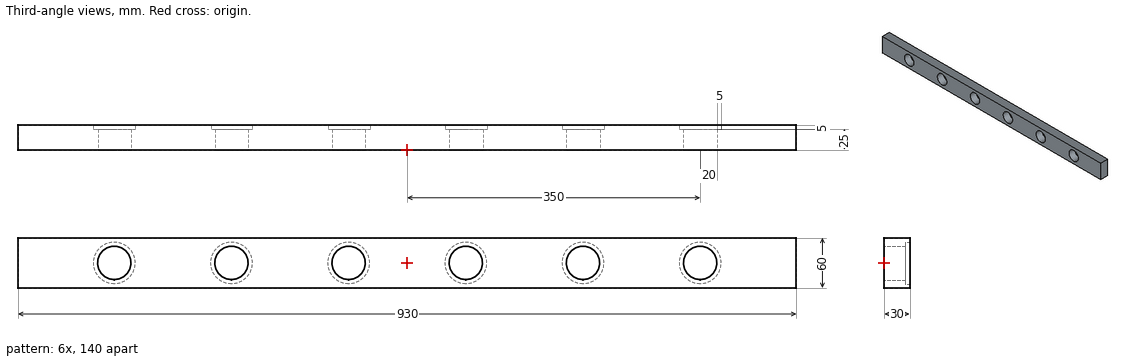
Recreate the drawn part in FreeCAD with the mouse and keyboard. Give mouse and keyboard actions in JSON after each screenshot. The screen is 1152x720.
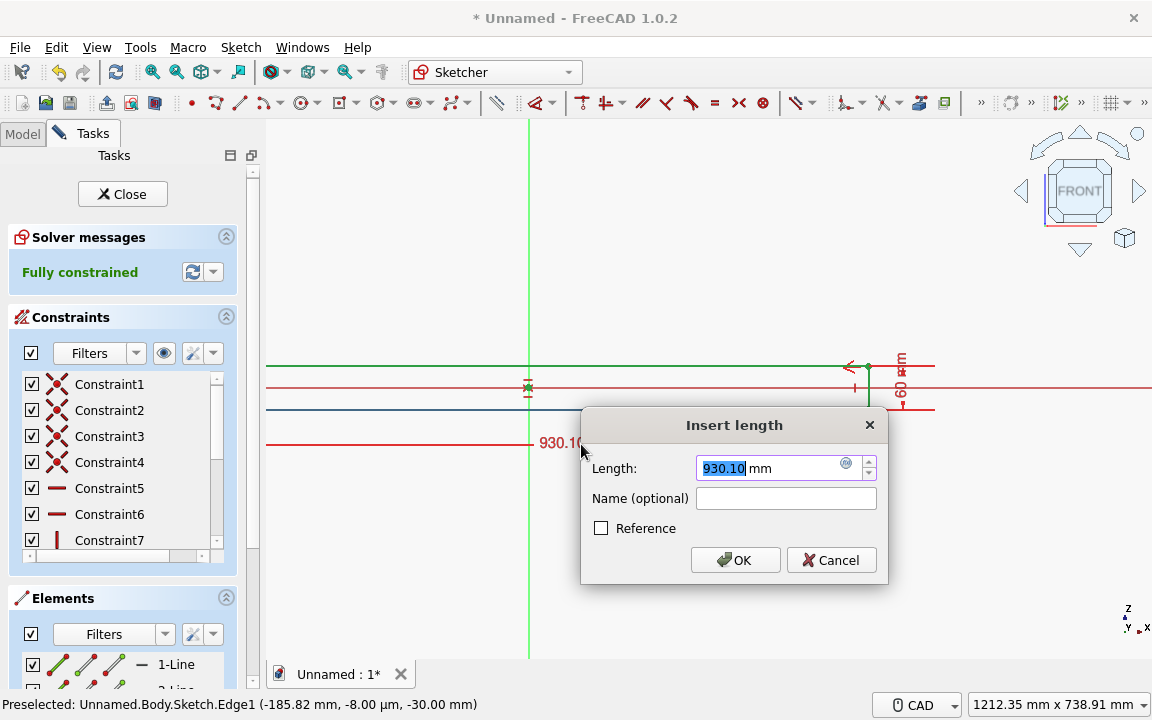
{"action": "type", "text": "930"}
{"action": "key", "text": "Return"}
{"action": "key", "text": "Escape"}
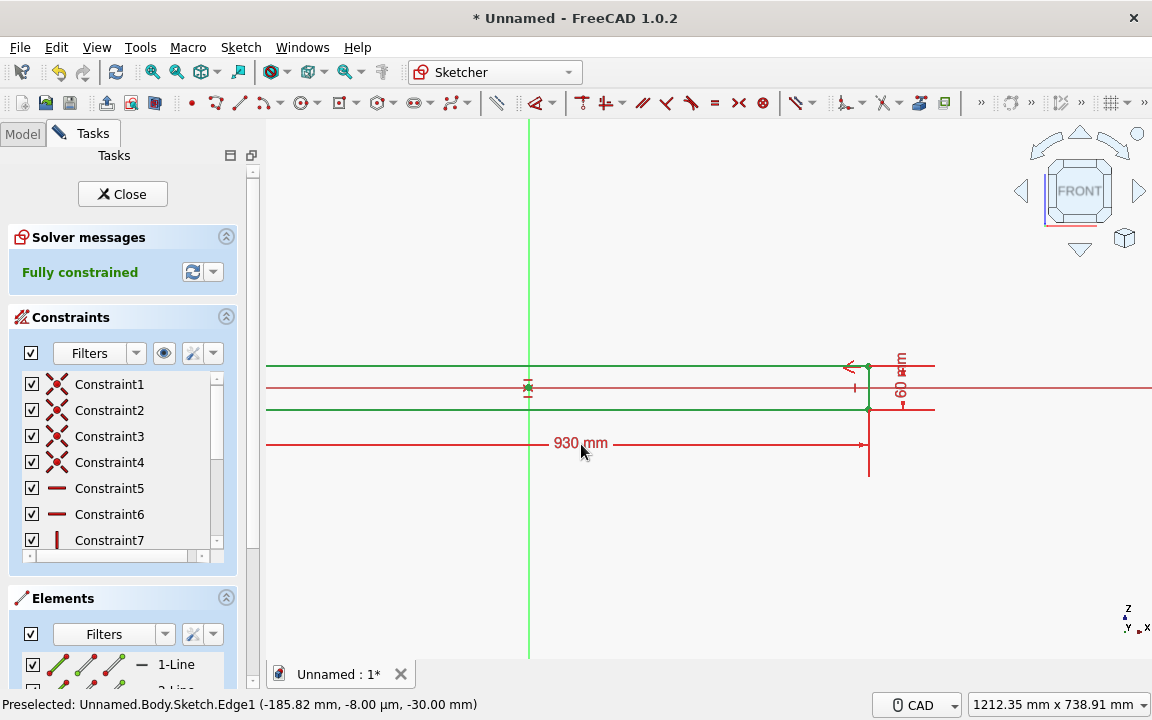
{"action": "left_click", "coordinate": [123, 194]}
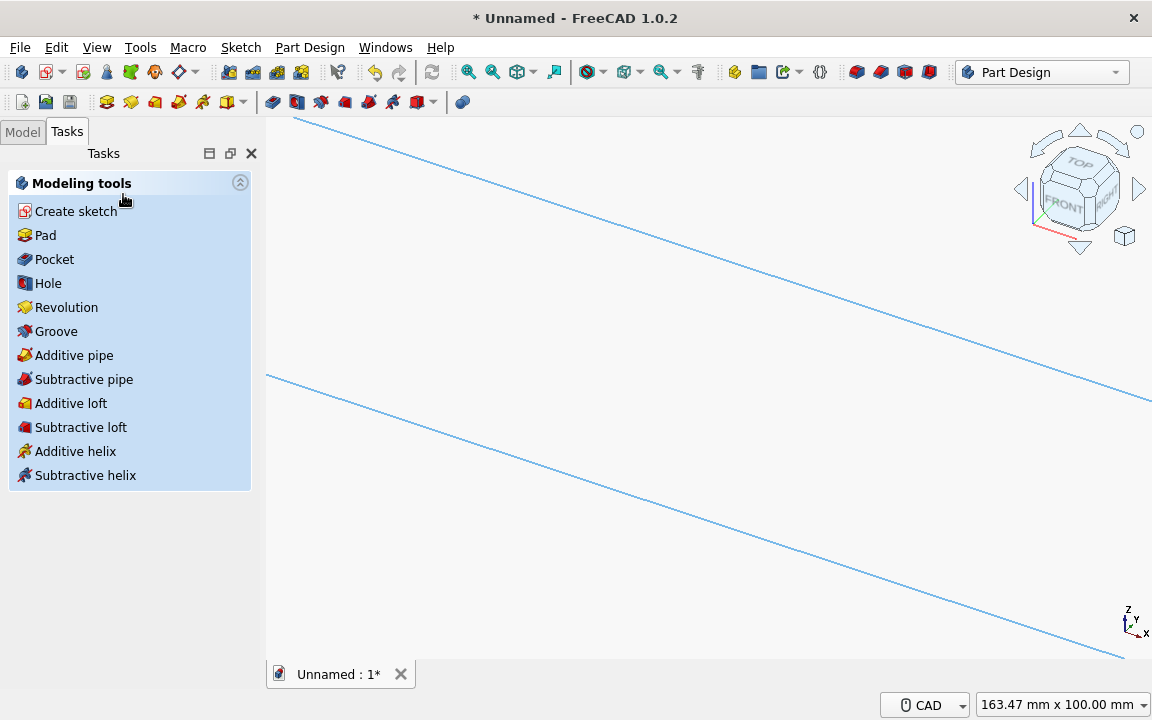
{"action": "left_click", "coordinate": [108, 102]}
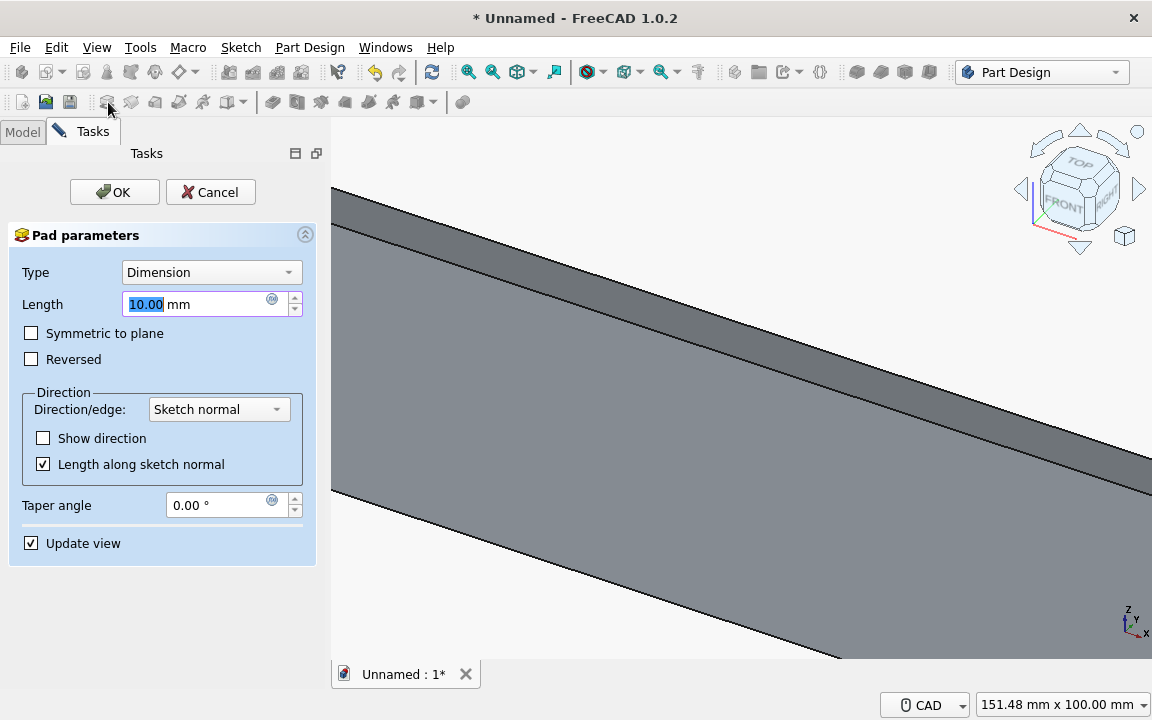
{"action": "type", "text": "30"}
{"action": "key", "text": "Tab"}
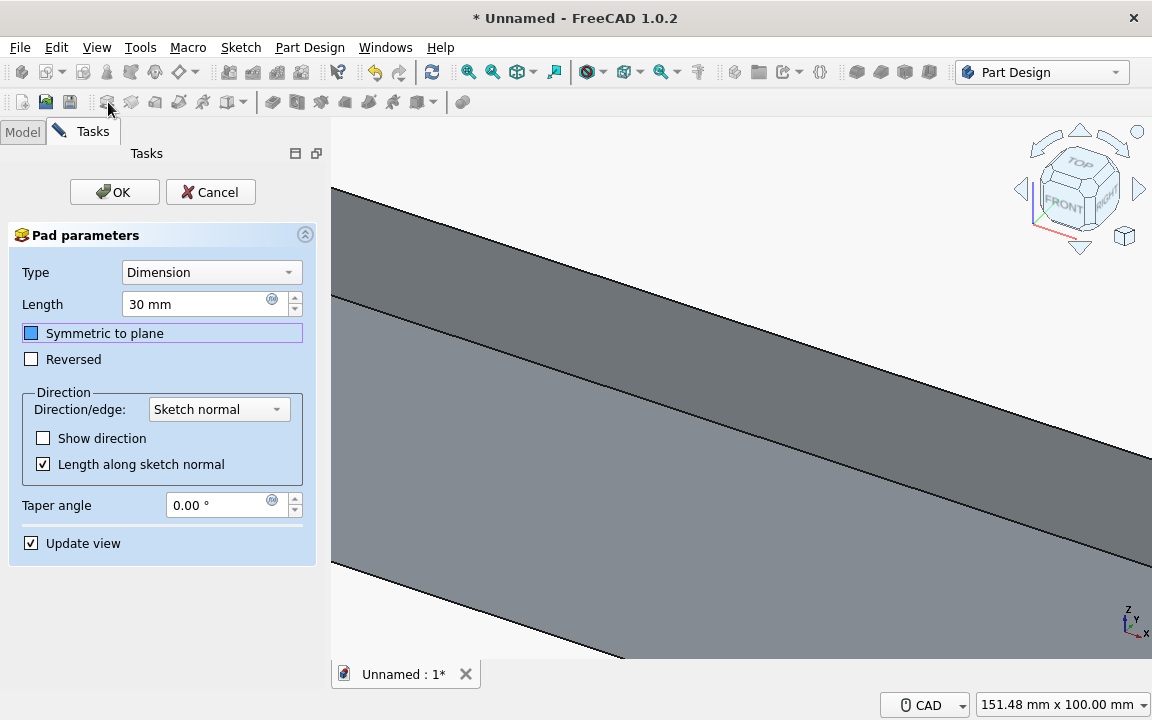
{"action": "left_click", "coordinate": [30, 359]}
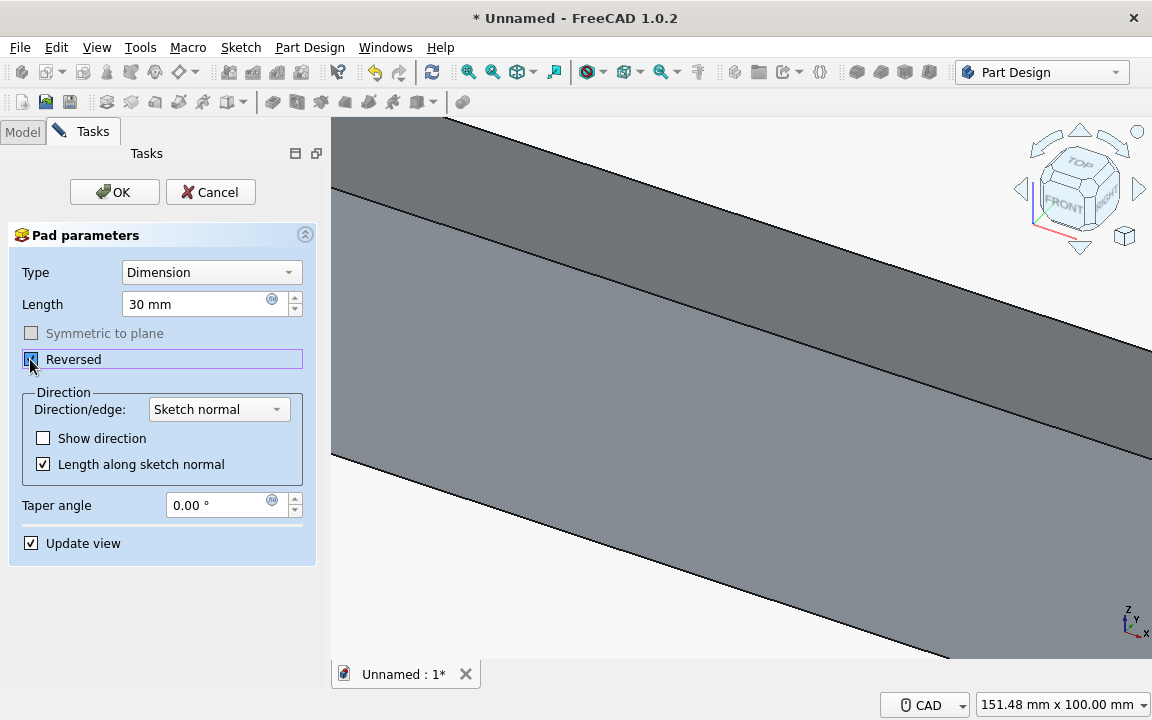
{"action": "left_click", "coordinate": [115, 192]}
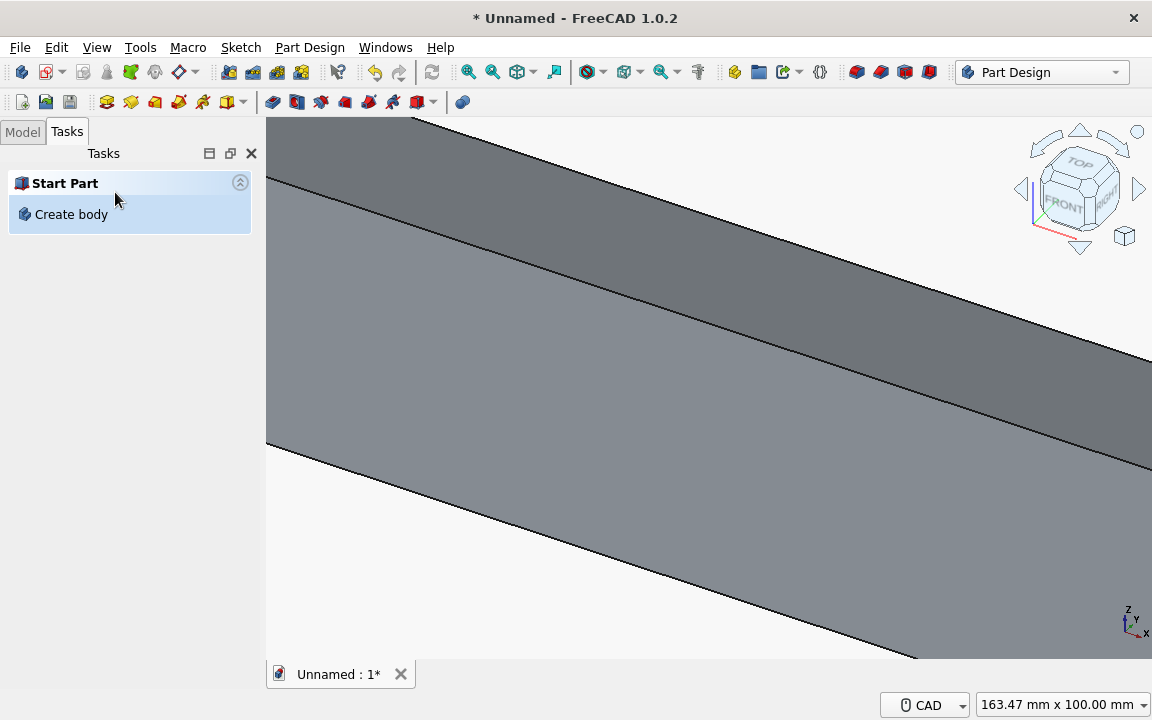
{"action": "left_click", "coordinate": [470, 72]}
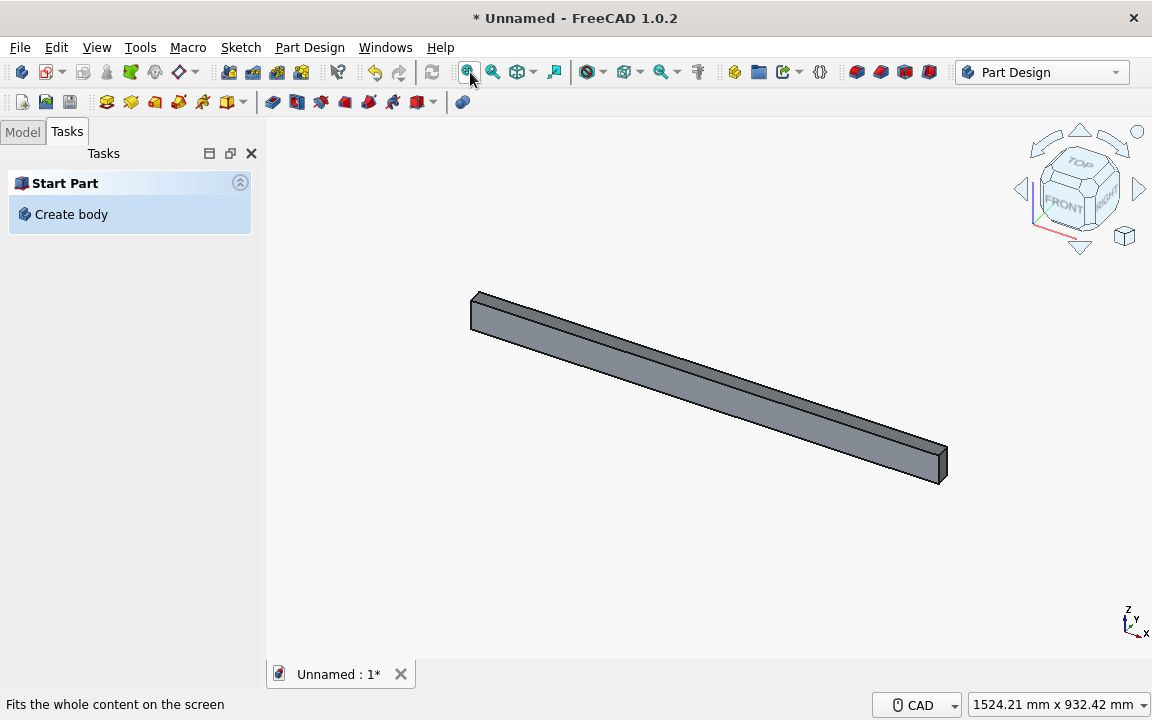
{"action": "left_click", "coordinate": [46, 72]}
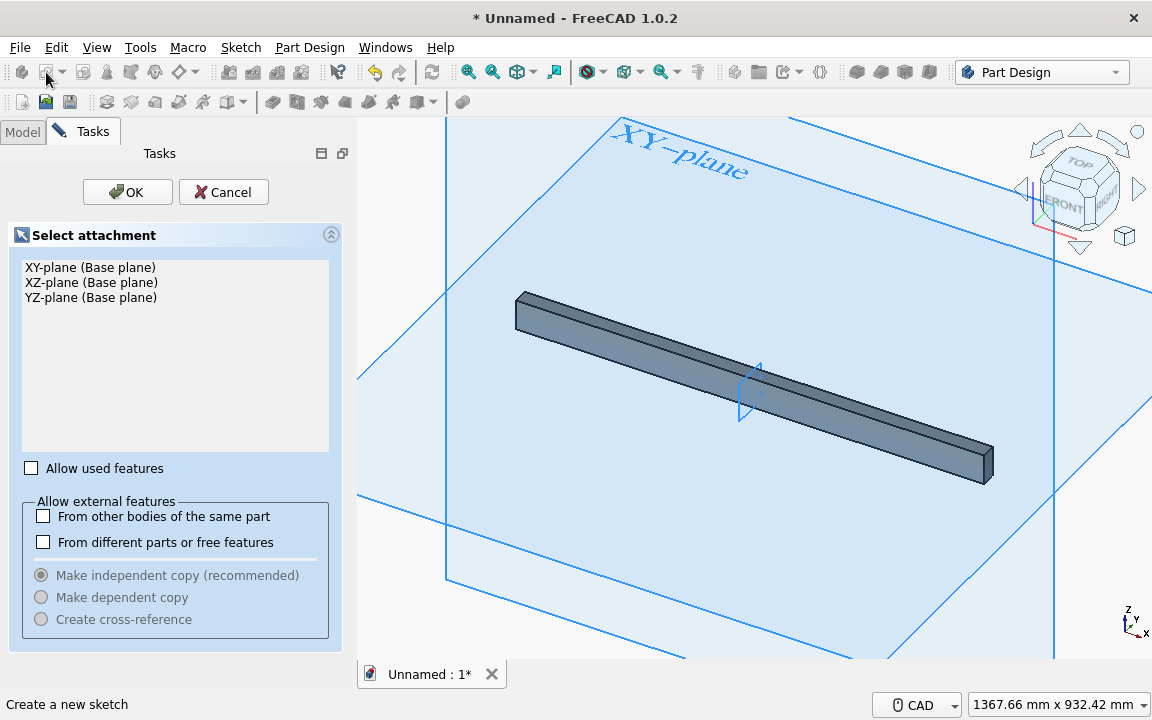
{"action": "left_click", "coordinate": [82, 268]}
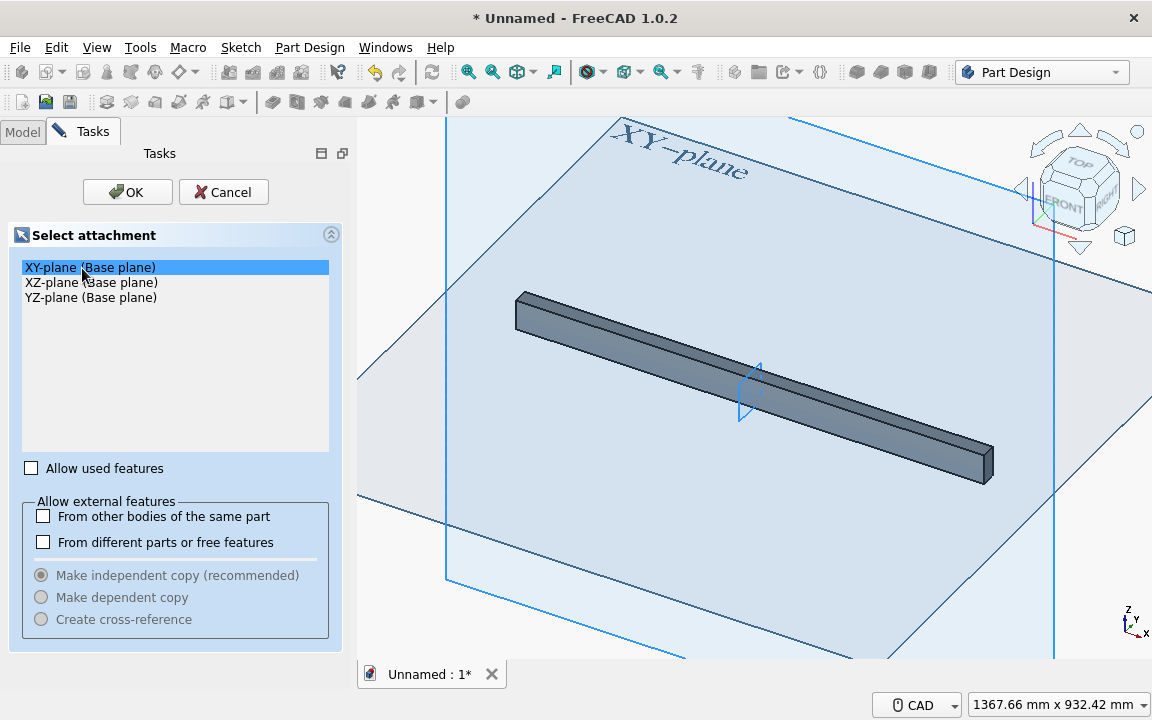
{"action": "left_click", "coordinate": [128, 192]}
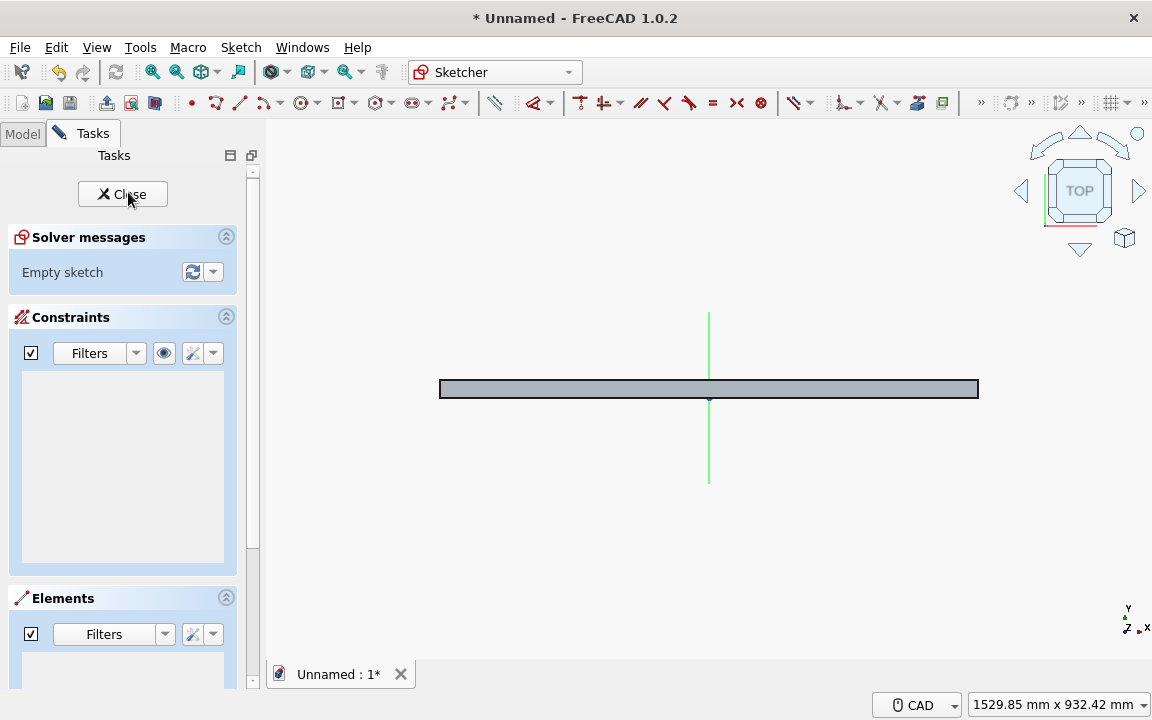
{"action": "left_click", "coordinate": [156, 104]}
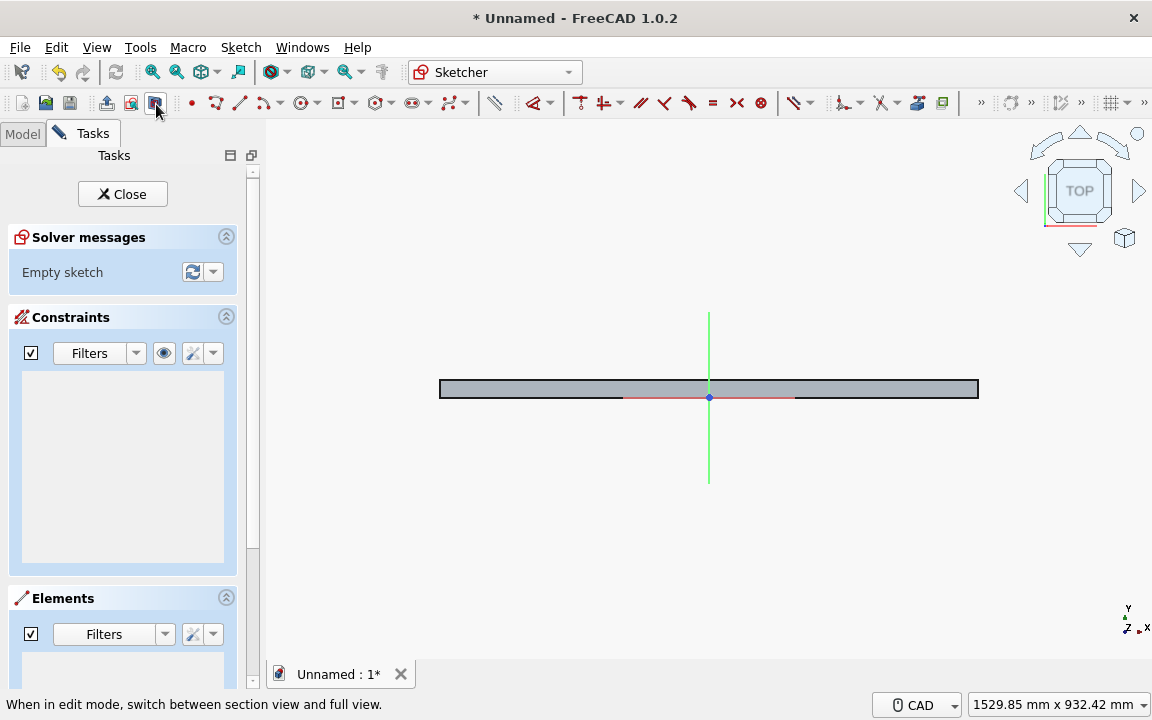
{"action": "scroll", "coordinate": [941, 385], "scroll_direction": "up", "scroll_amount": 13}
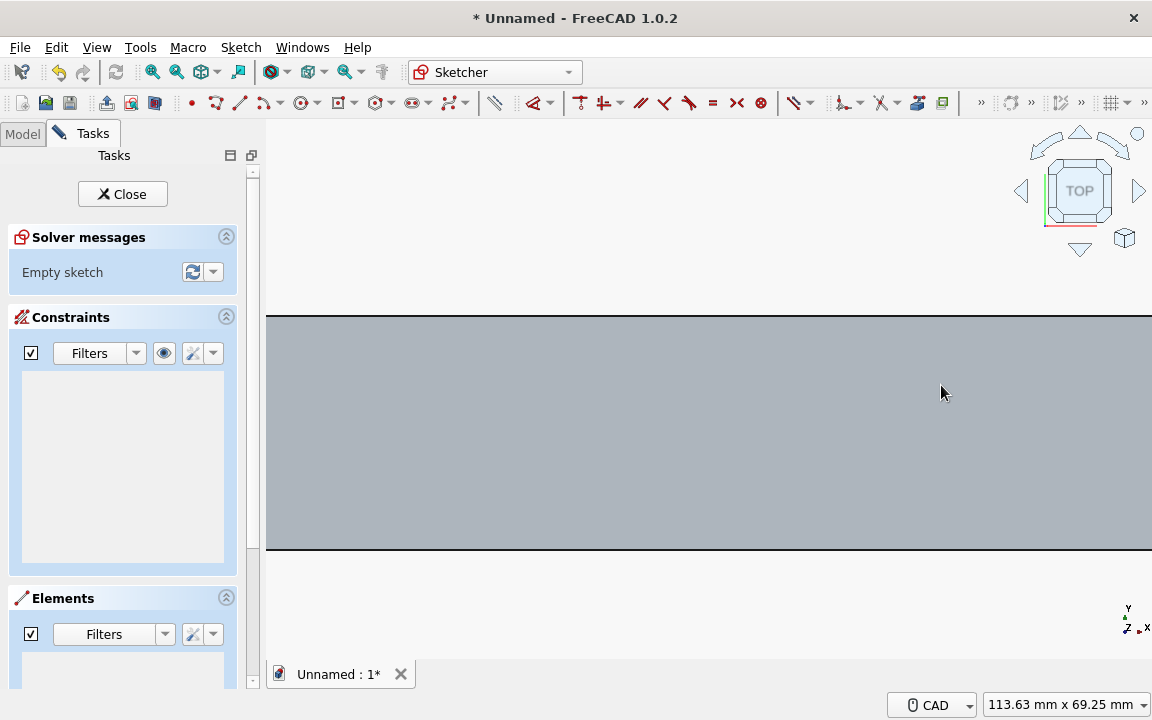
{"action": "key", "text": "g m"}